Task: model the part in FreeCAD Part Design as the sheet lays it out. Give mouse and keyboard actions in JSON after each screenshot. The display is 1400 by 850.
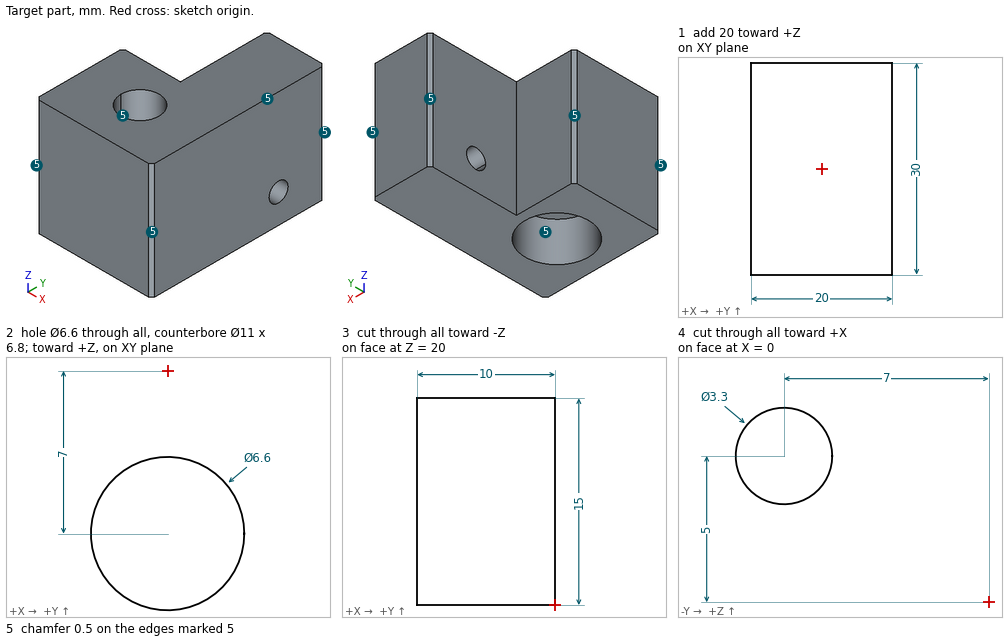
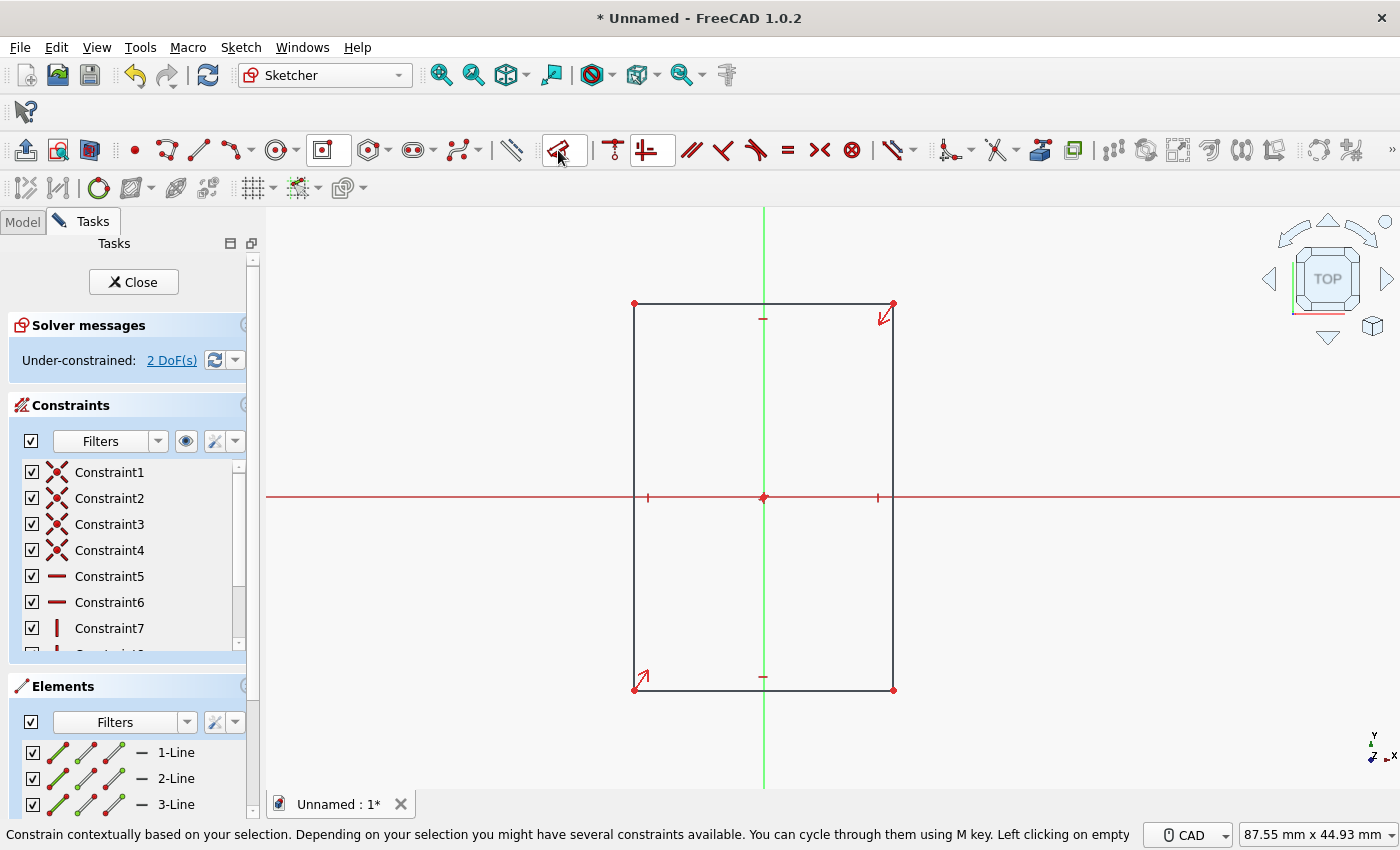
{"action": "left_click", "coordinate": [712, 691]}
{"action": "left_click", "coordinate": [704, 725]}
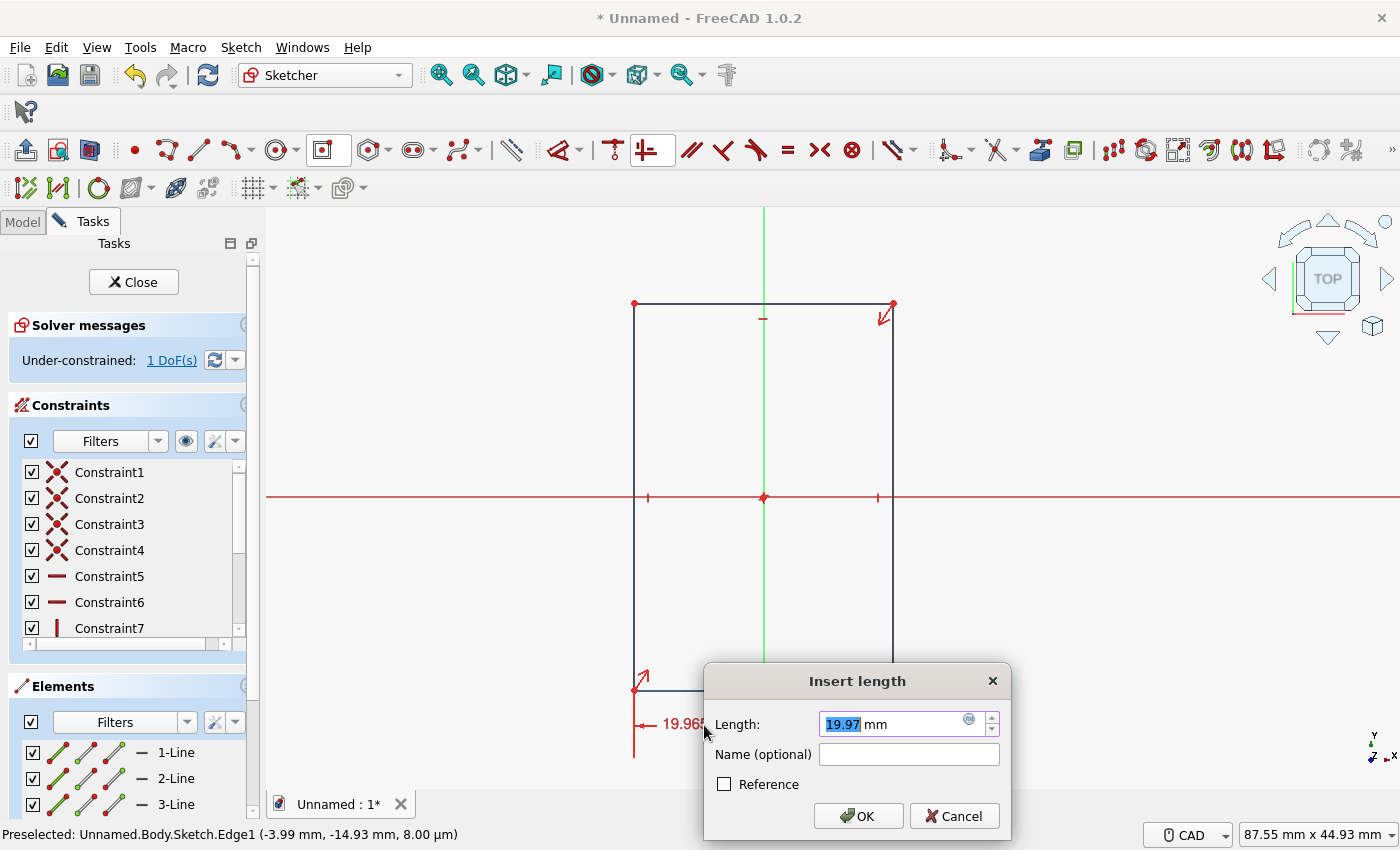
{"action": "type", "text": "20"}
{"action": "key", "text": "Return"}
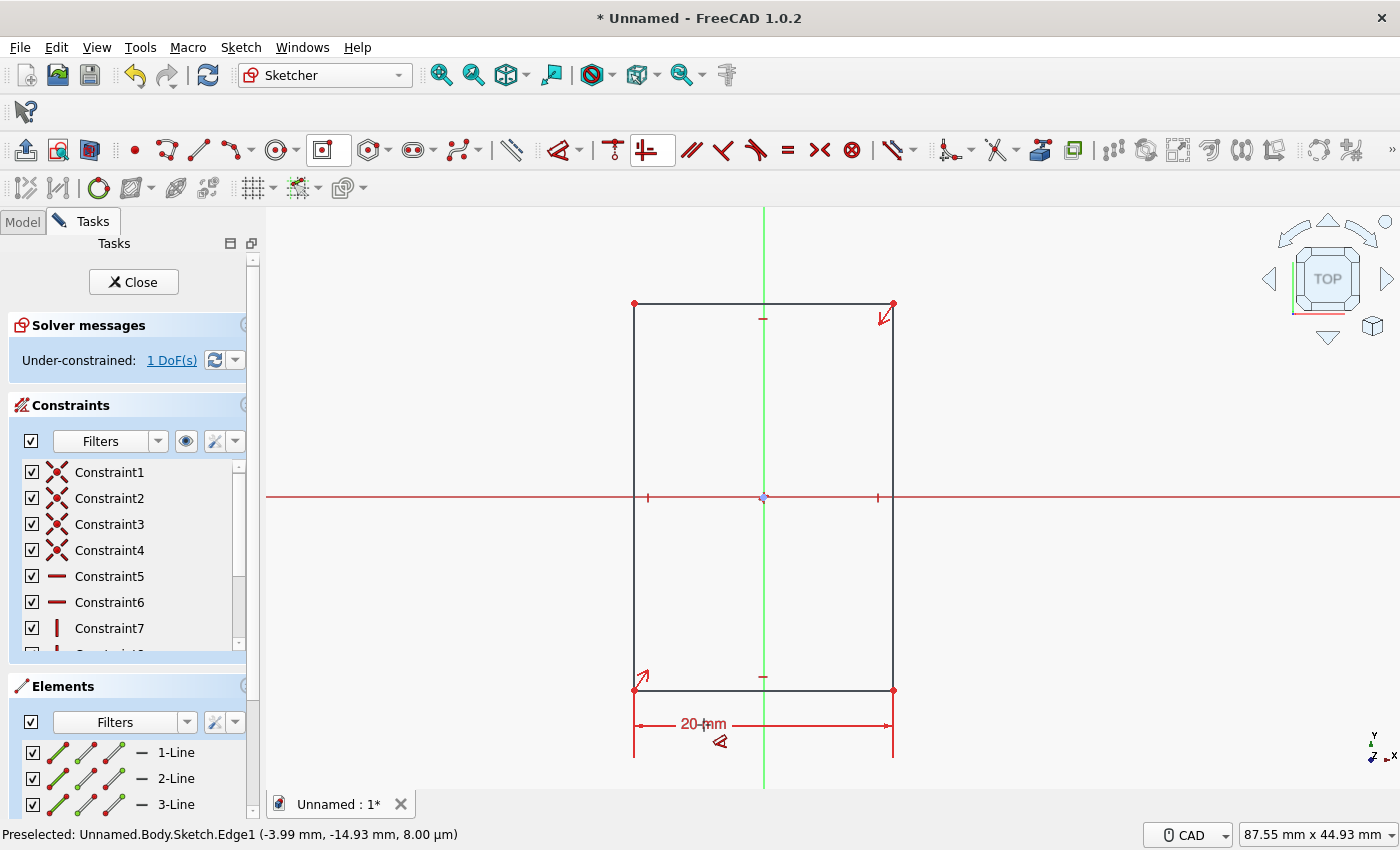
{"action": "left_click", "coordinate": [893, 575]}
{"action": "left_click", "coordinate": [927, 408]}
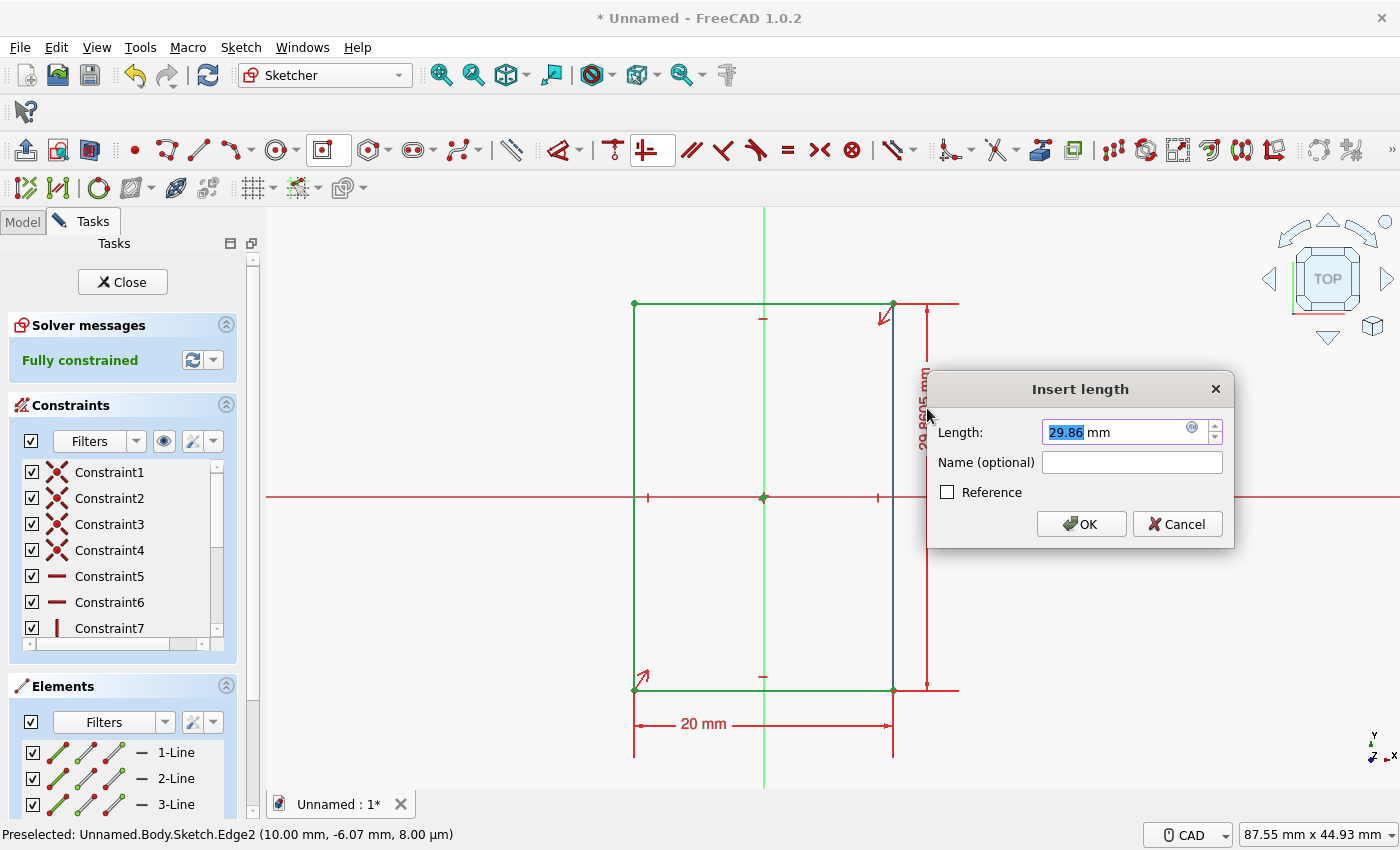
{"action": "type", "text": "30"}
{"action": "key", "text": "Return"}
{"action": "key", "text": "Escape"}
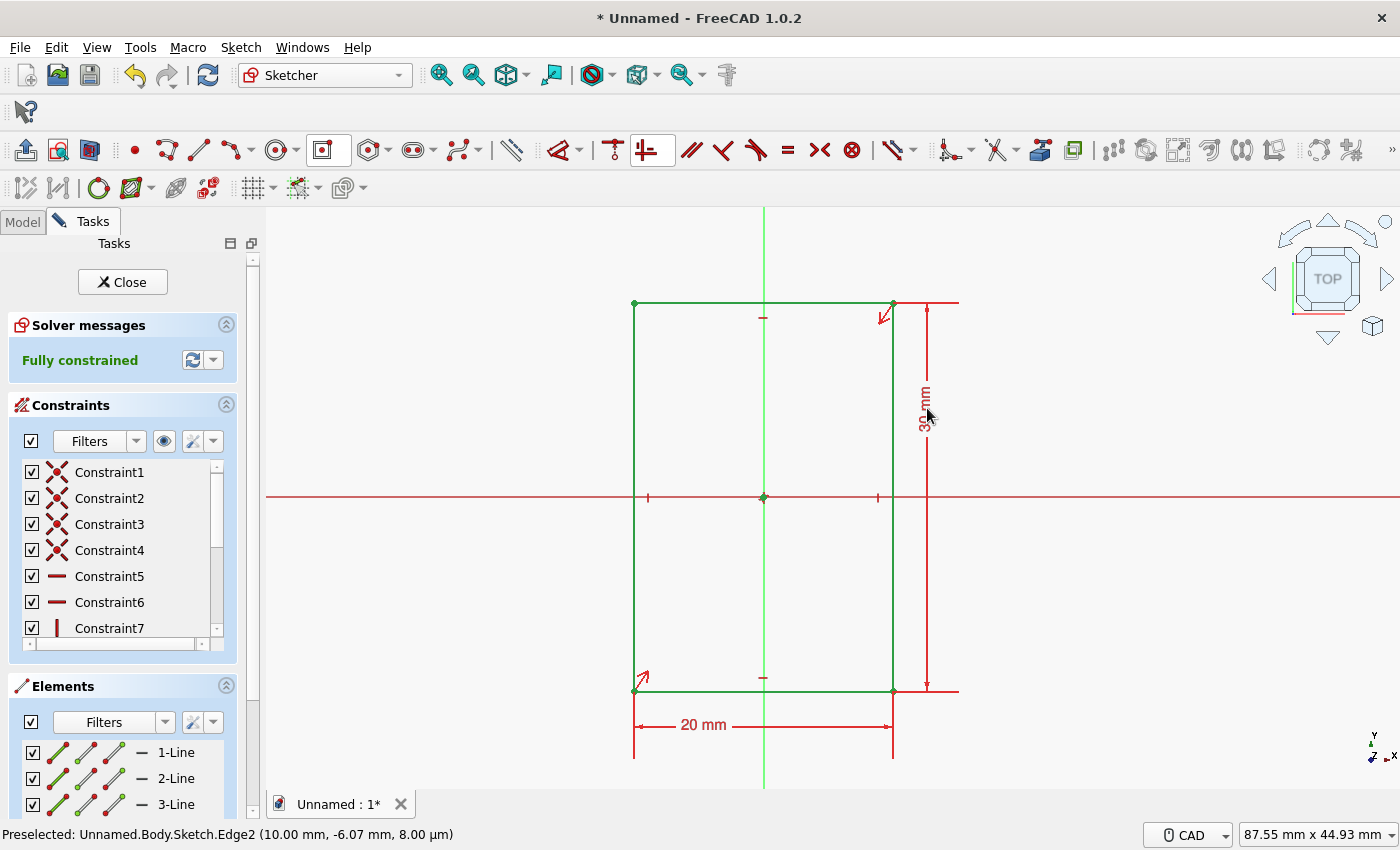
{"action": "left_click", "coordinate": [123, 282]}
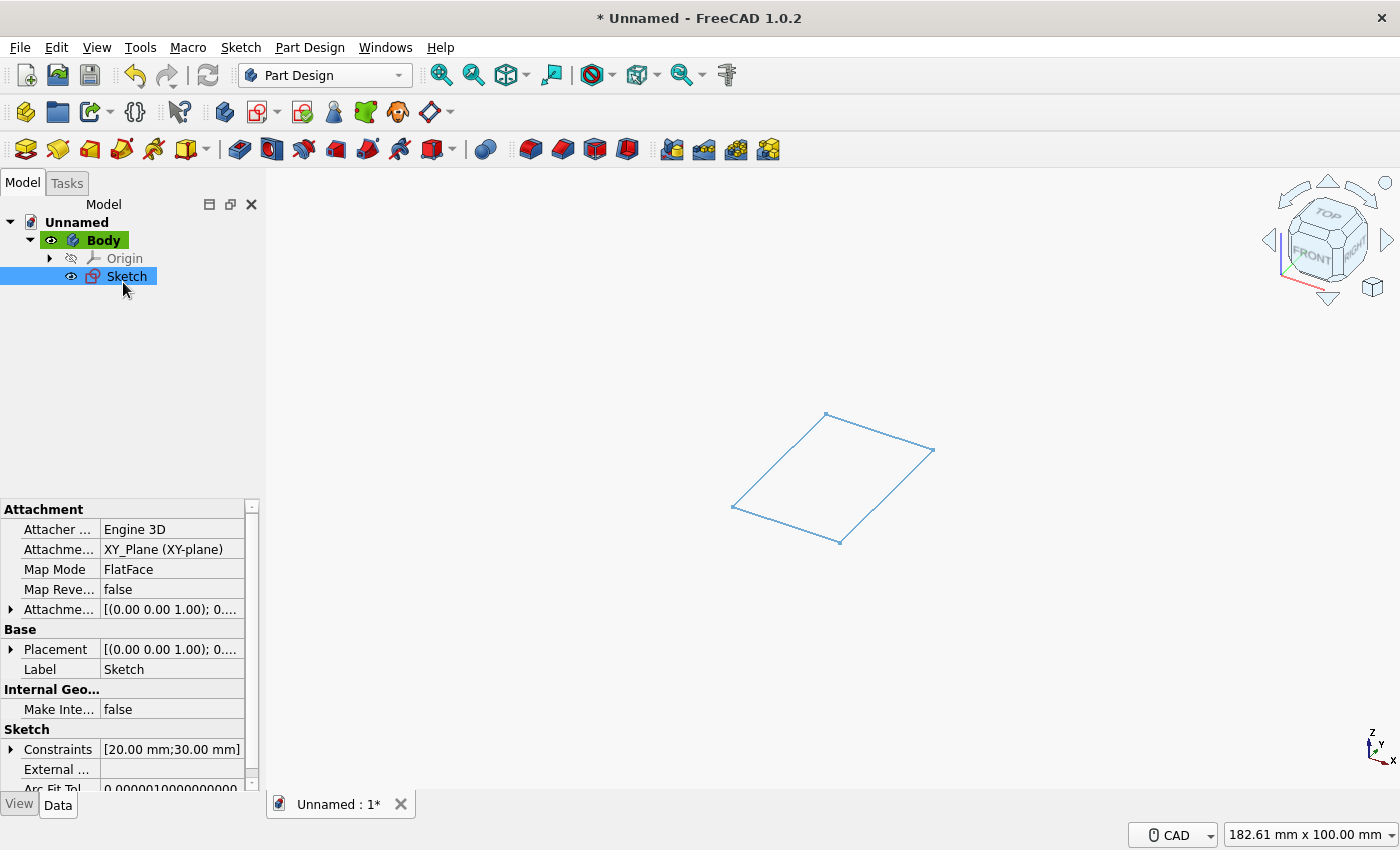
{"action": "left_click", "coordinate": [26, 150]}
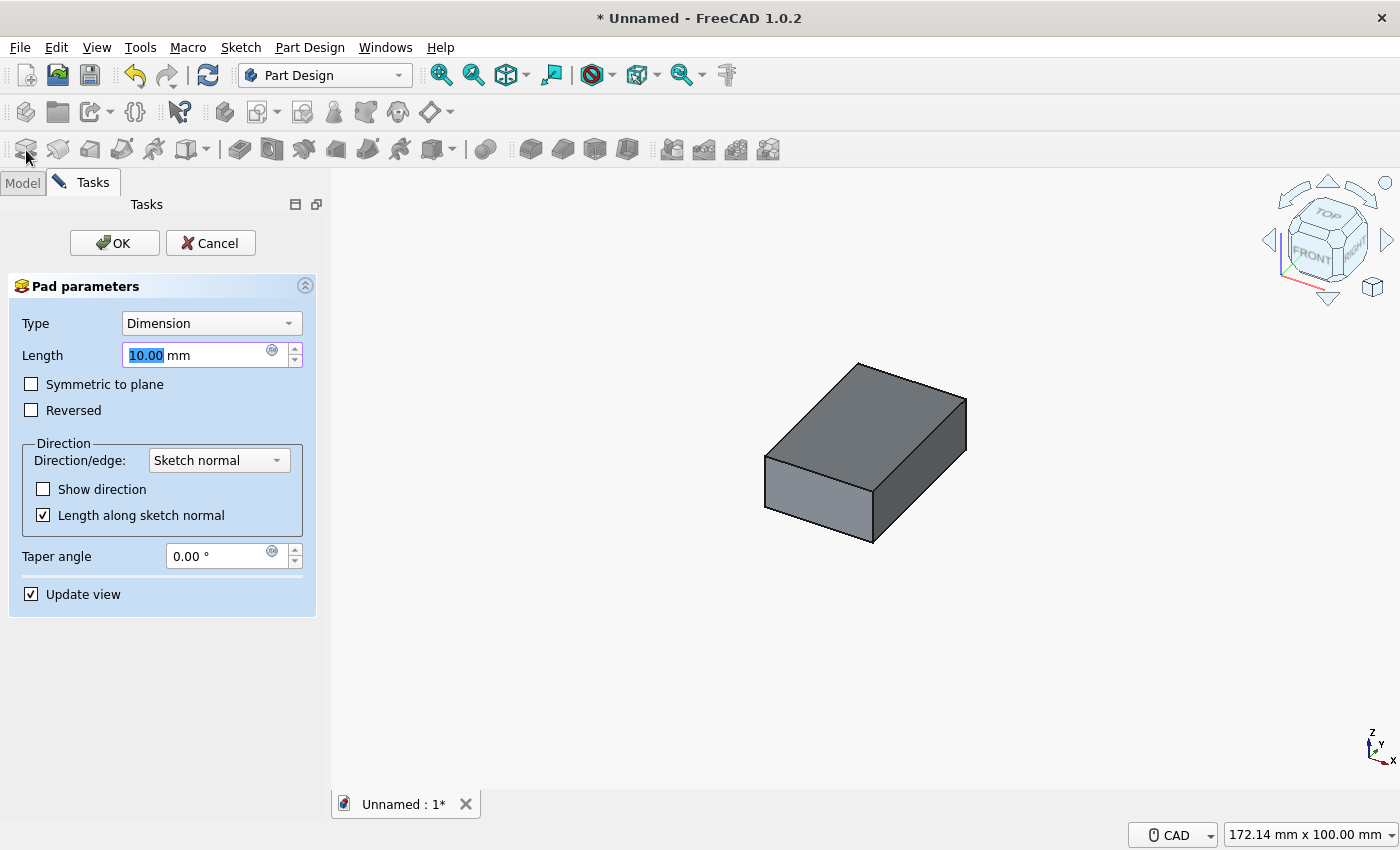
{"action": "type", "text": "20"}
{"action": "key", "text": "Tab"}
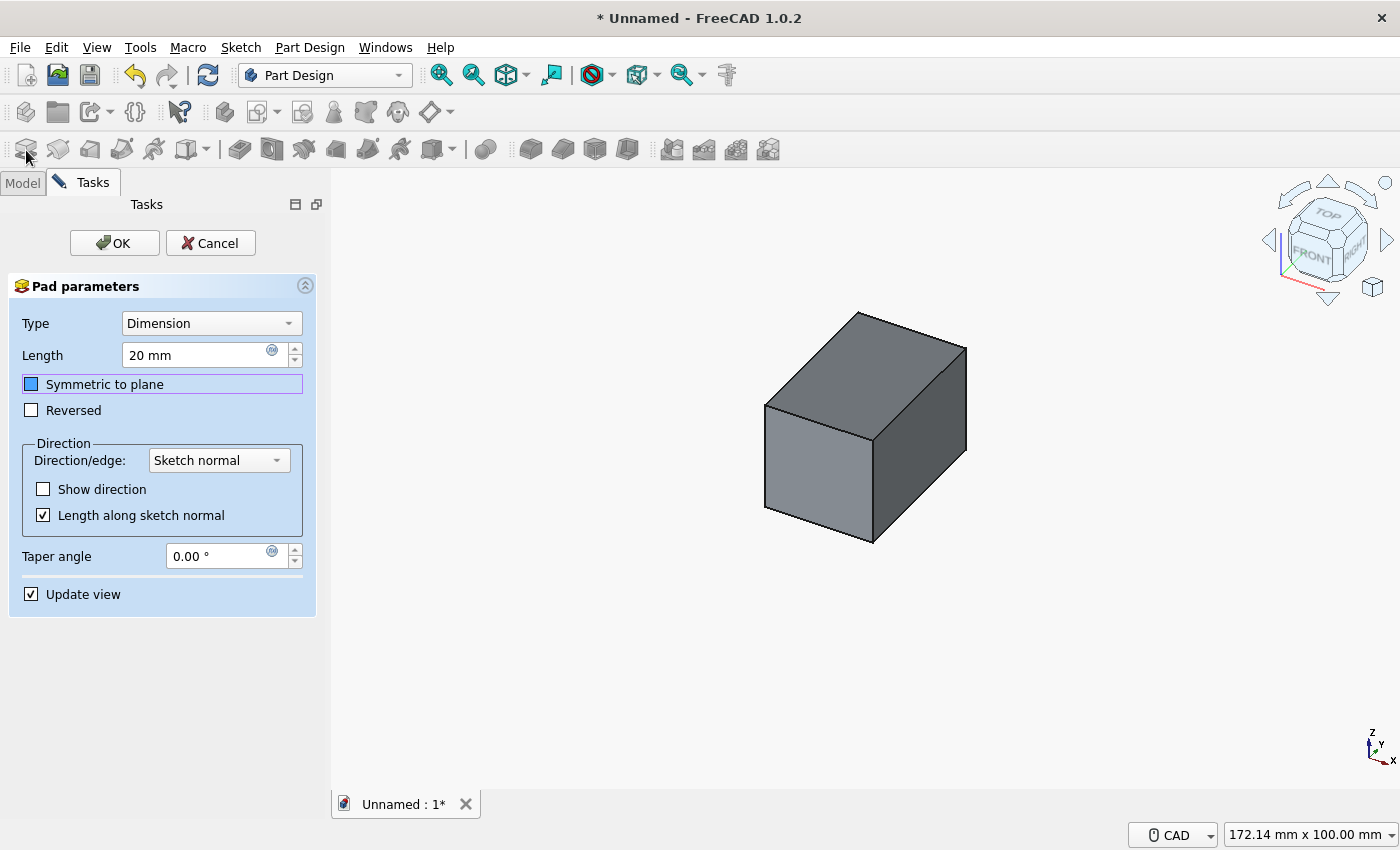
{"action": "left_click", "coordinate": [115, 243]}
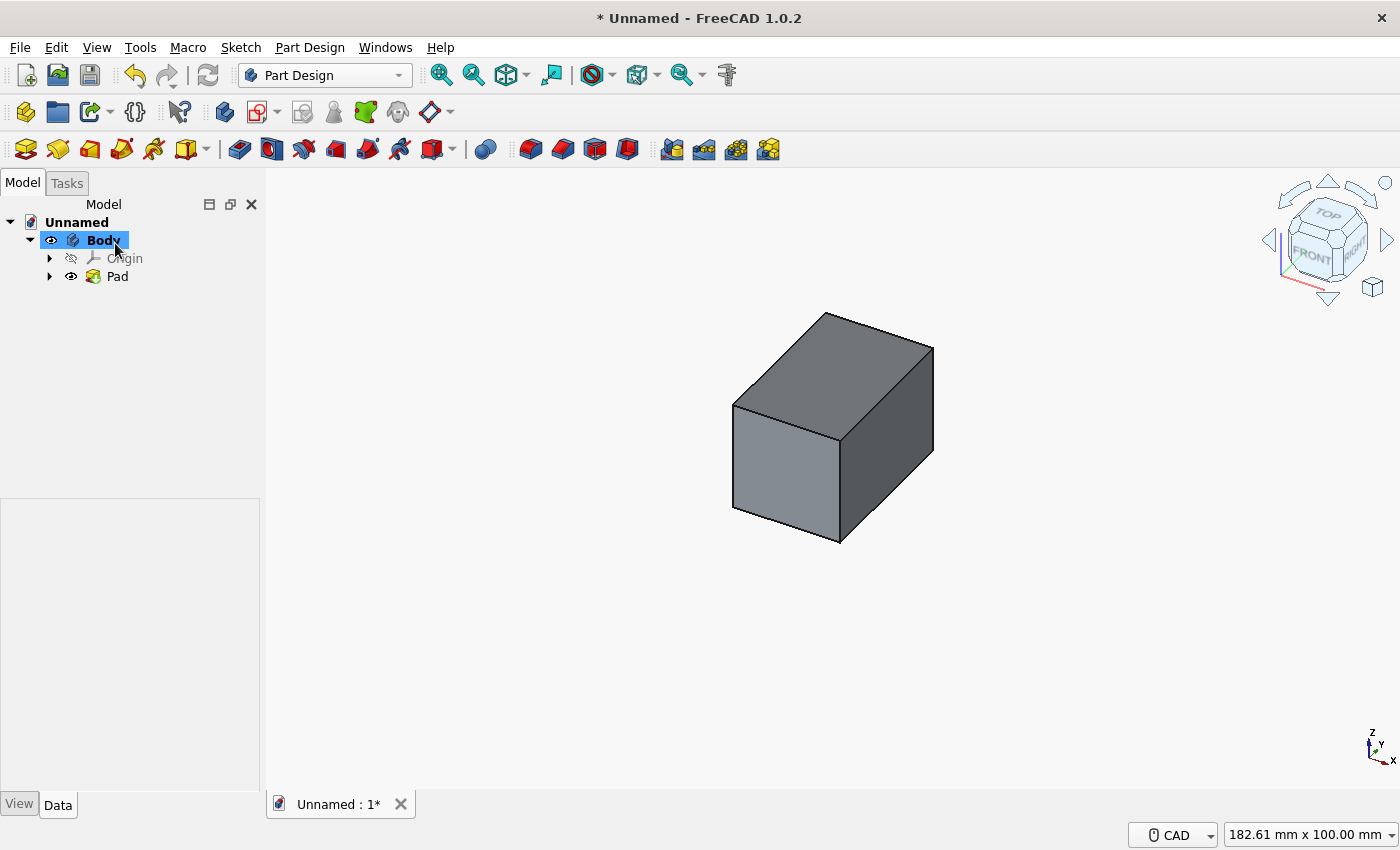
{"action": "left_click", "coordinate": [442, 76]}